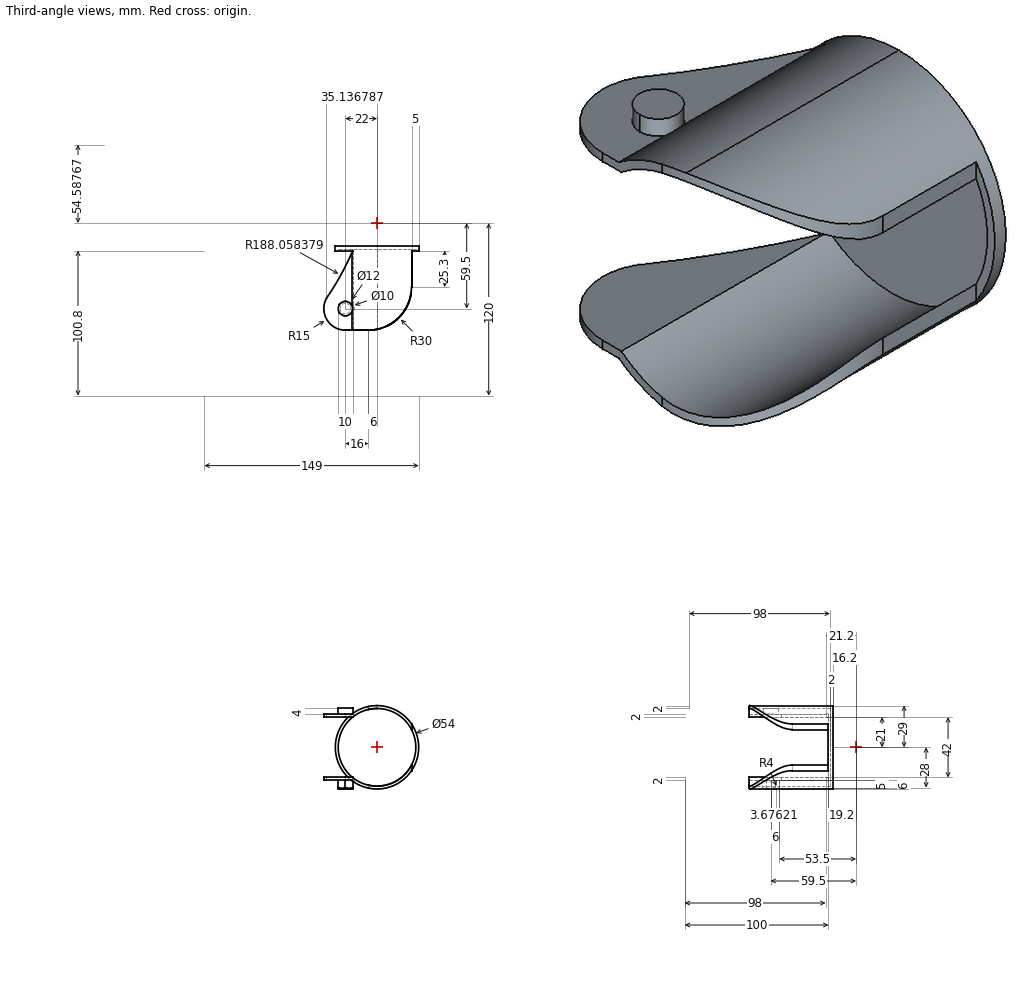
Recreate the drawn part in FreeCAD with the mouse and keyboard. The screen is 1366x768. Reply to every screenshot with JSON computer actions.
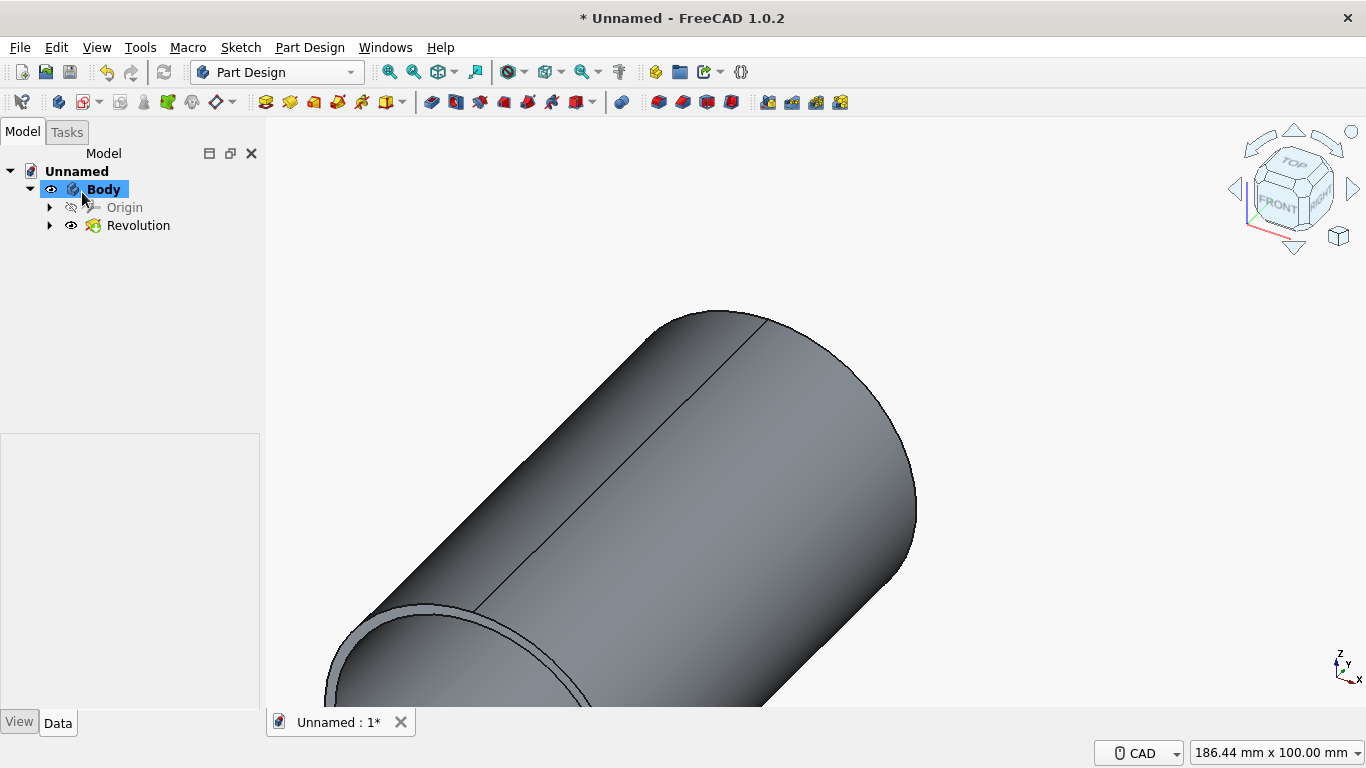
{"action": "key", "text": "v f"}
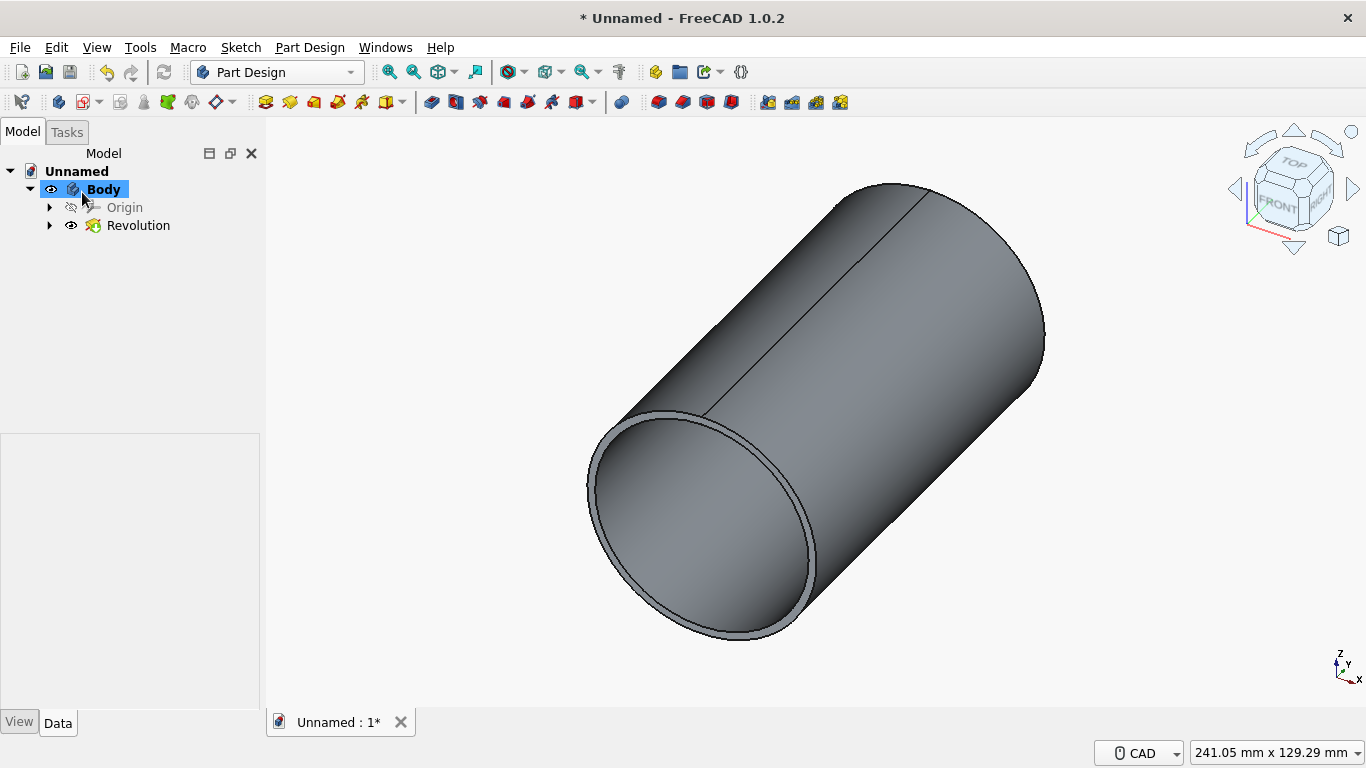
{"action": "left_click", "coordinate": [84, 102]}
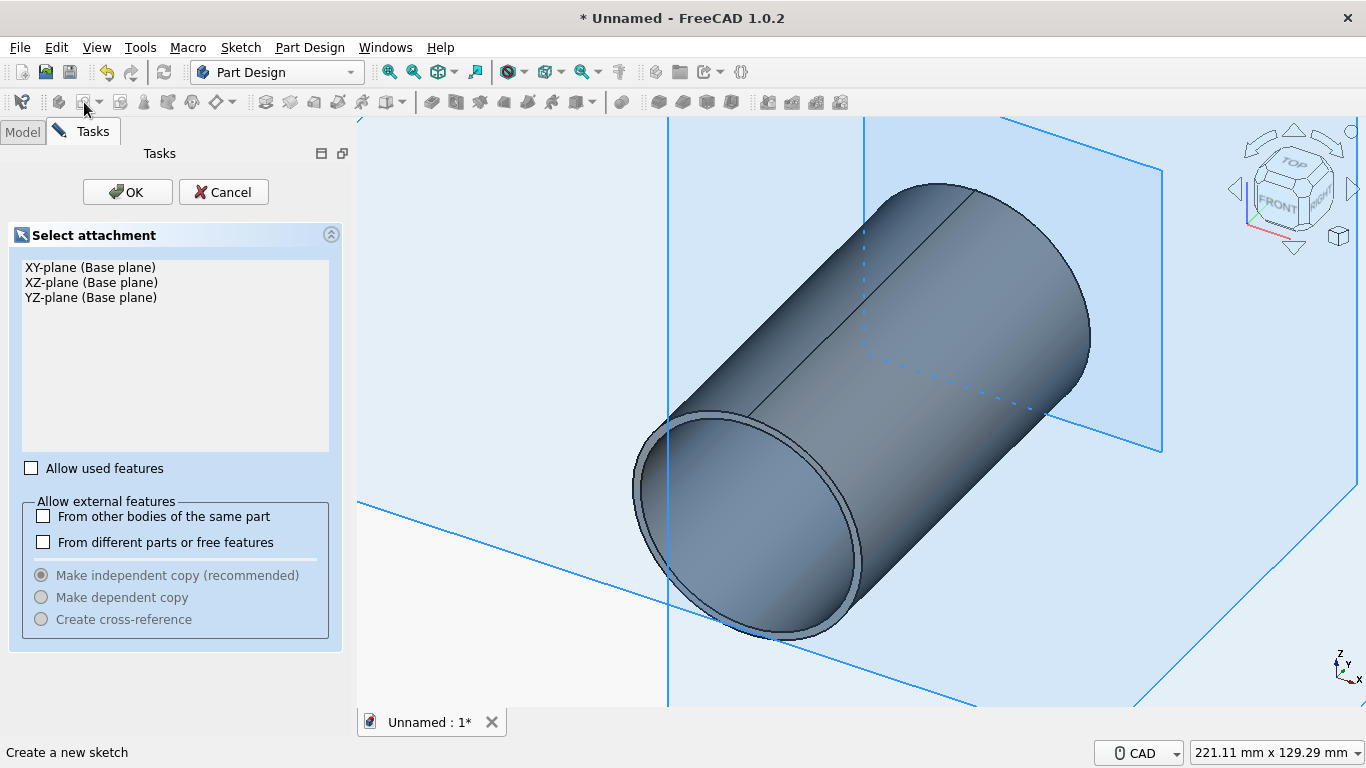
{"action": "left_click", "coordinate": [82, 298]}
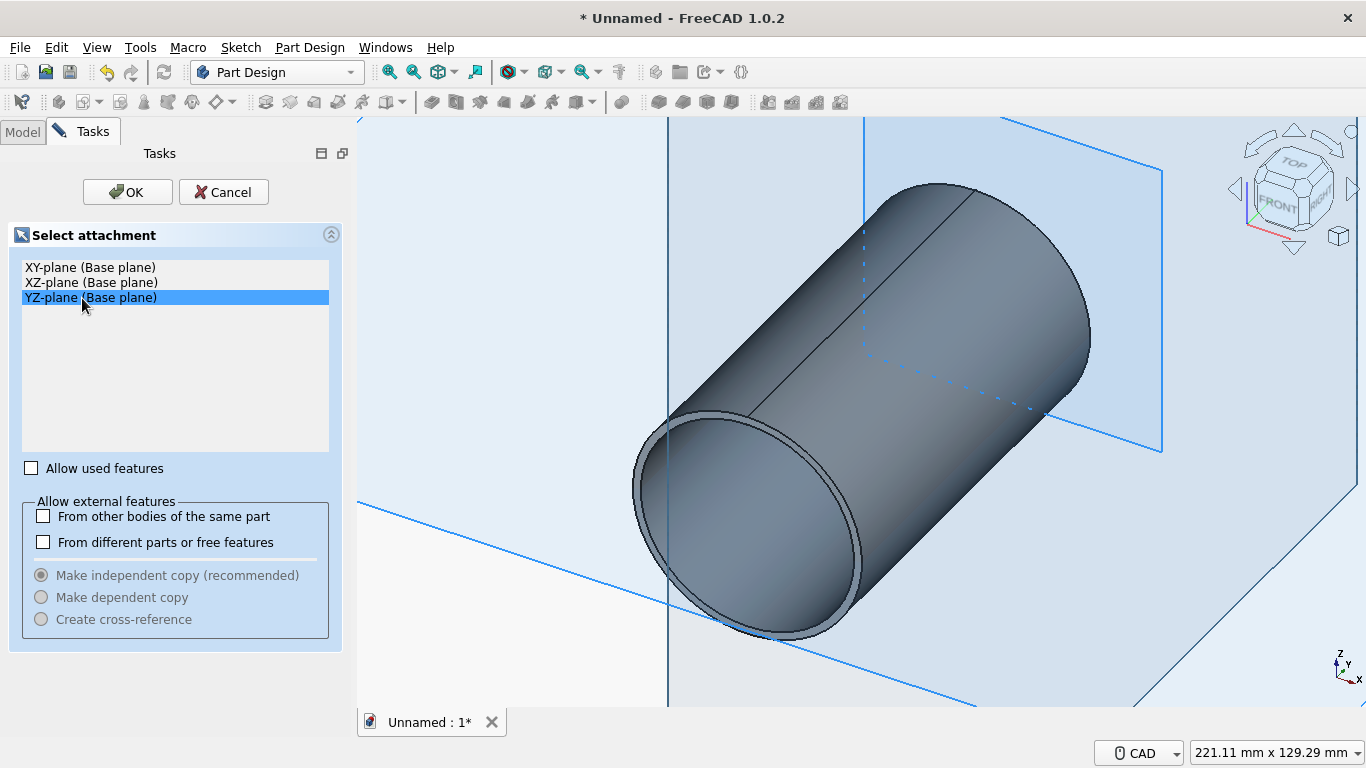
{"action": "left_click", "coordinate": [128, 192]}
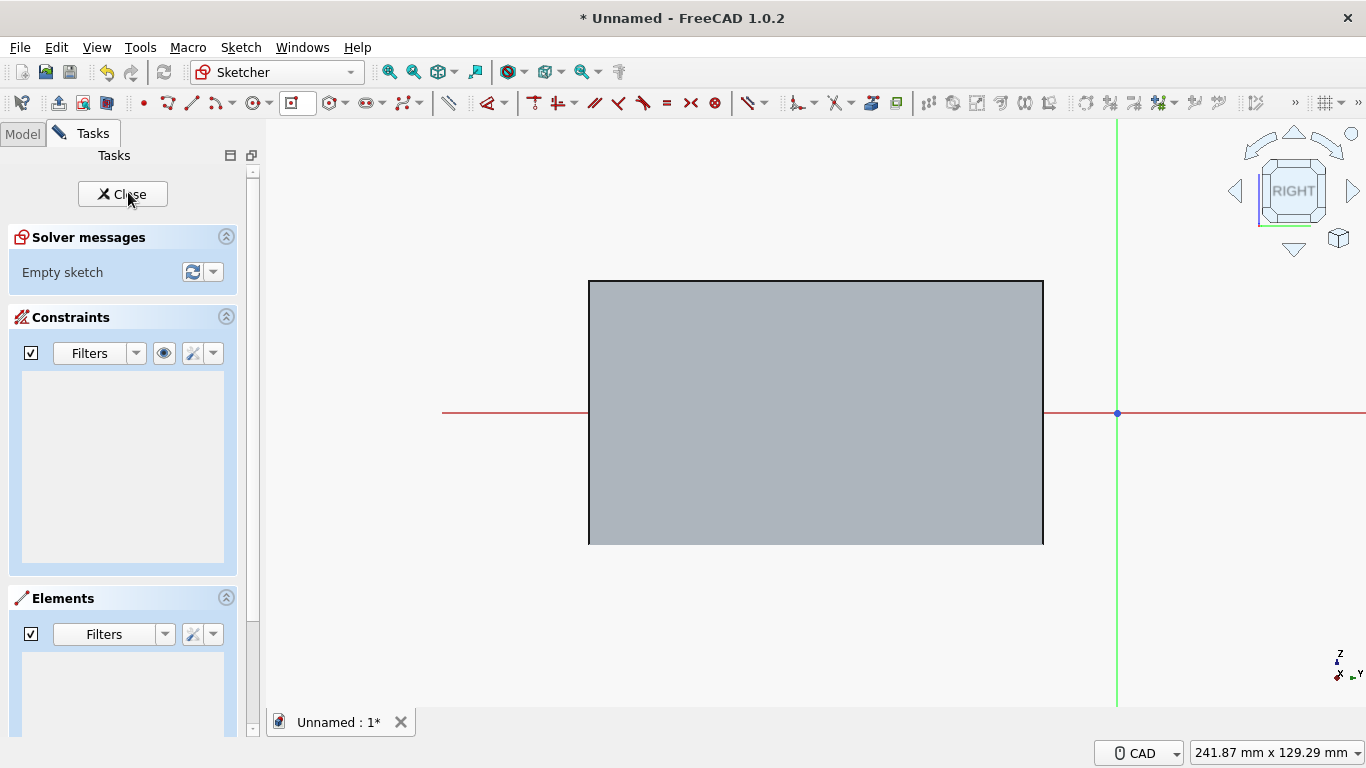
{"action": "key", "text": "q s"}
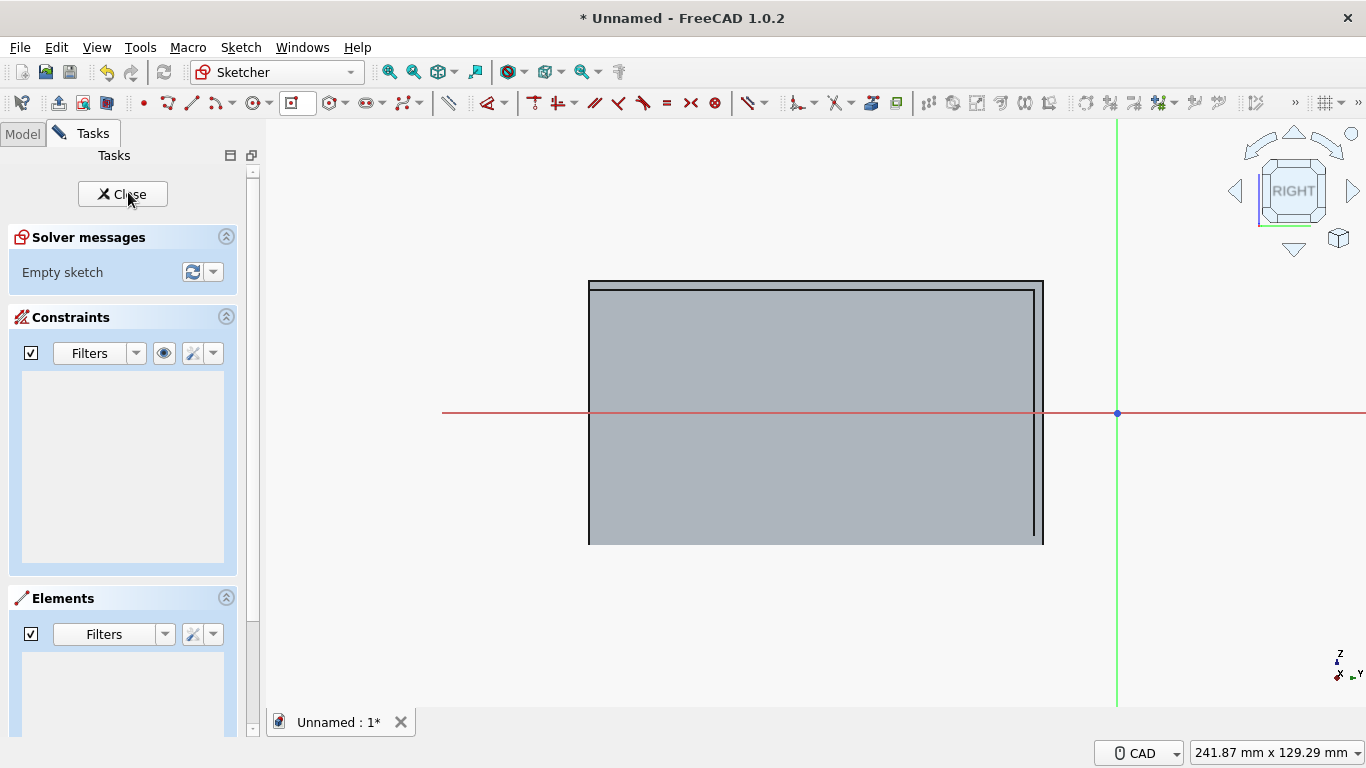
{"action": "key", "text": "g m"}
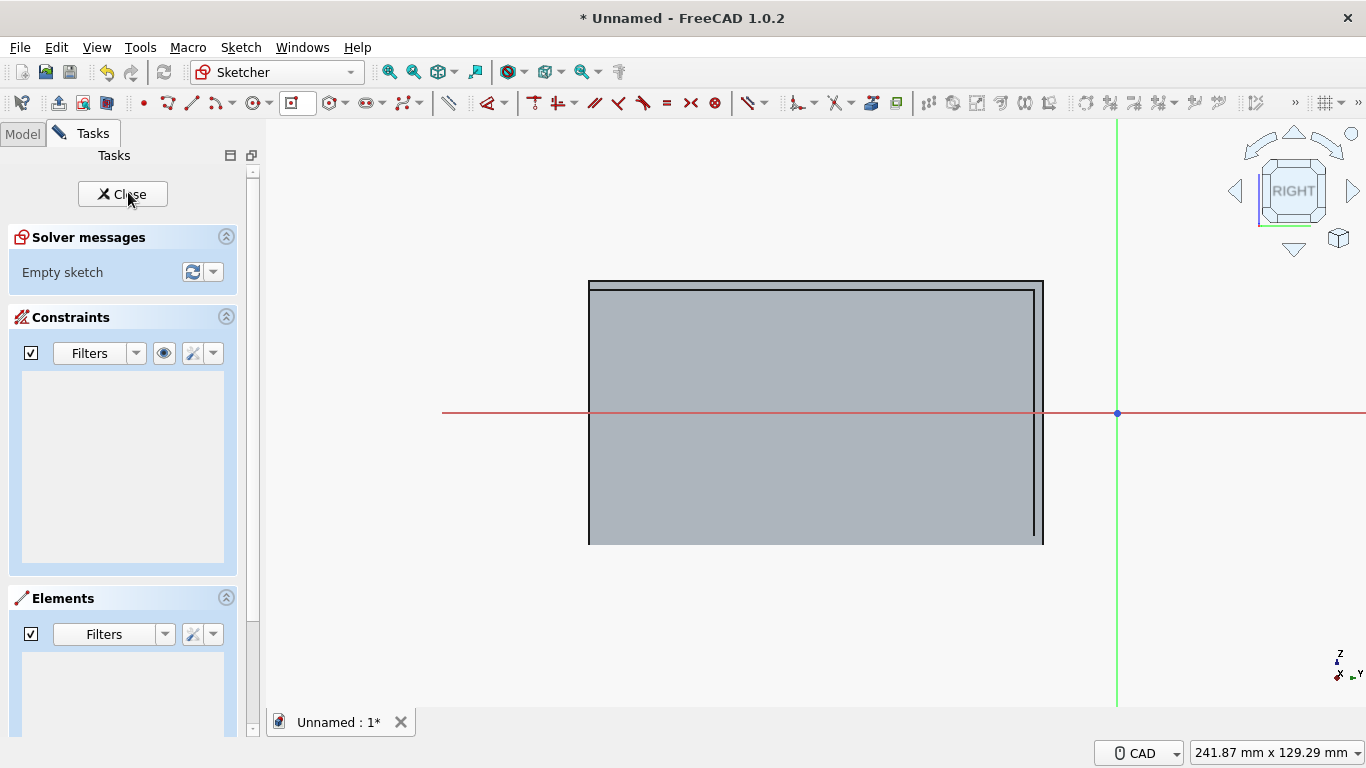
{"action": "left_click", "coordinate": [1021, 318]}
{"action": "left_click", "coordinate": [1021, 509]}
{"action": "left_click", "coordinate": [575, 509]}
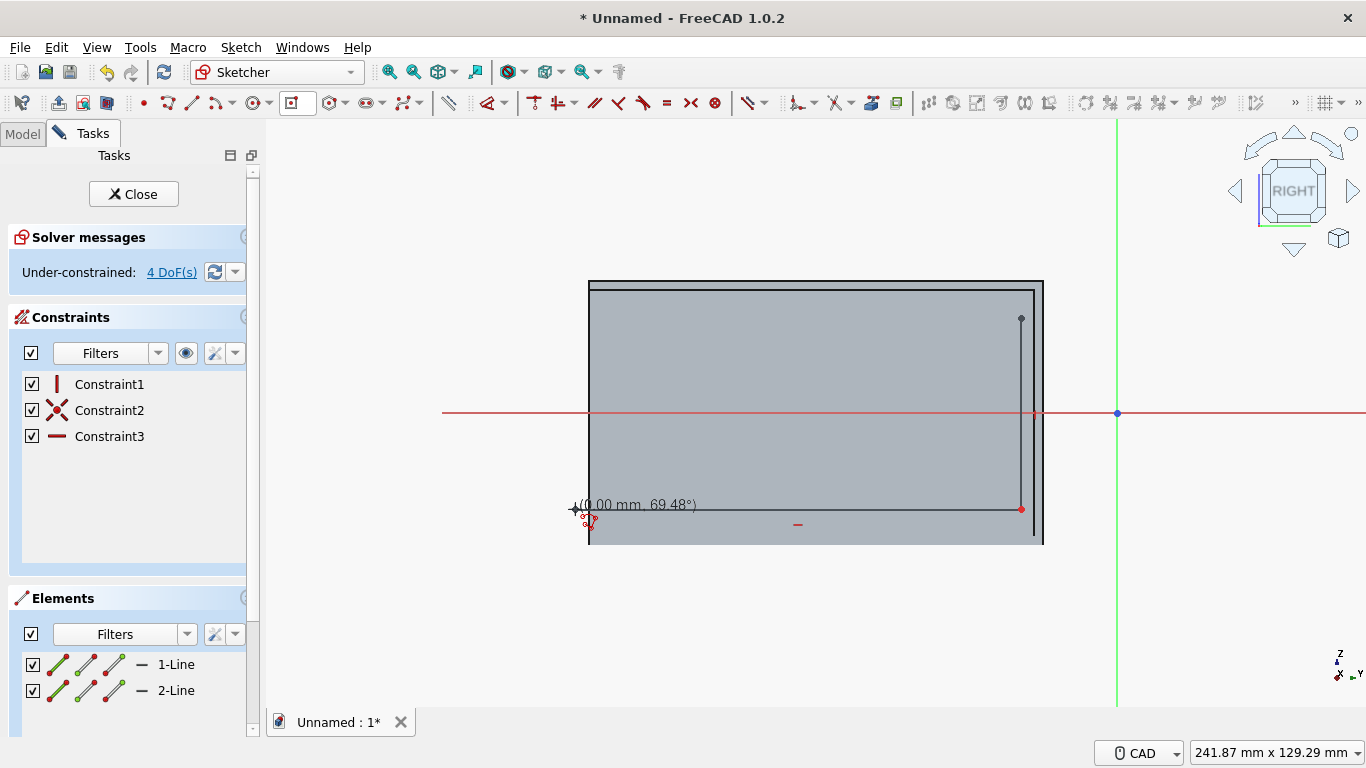
{"action": "scroll", "coordinate": [575, 518], "scroll_direction": "up", "scroll_amount": 3}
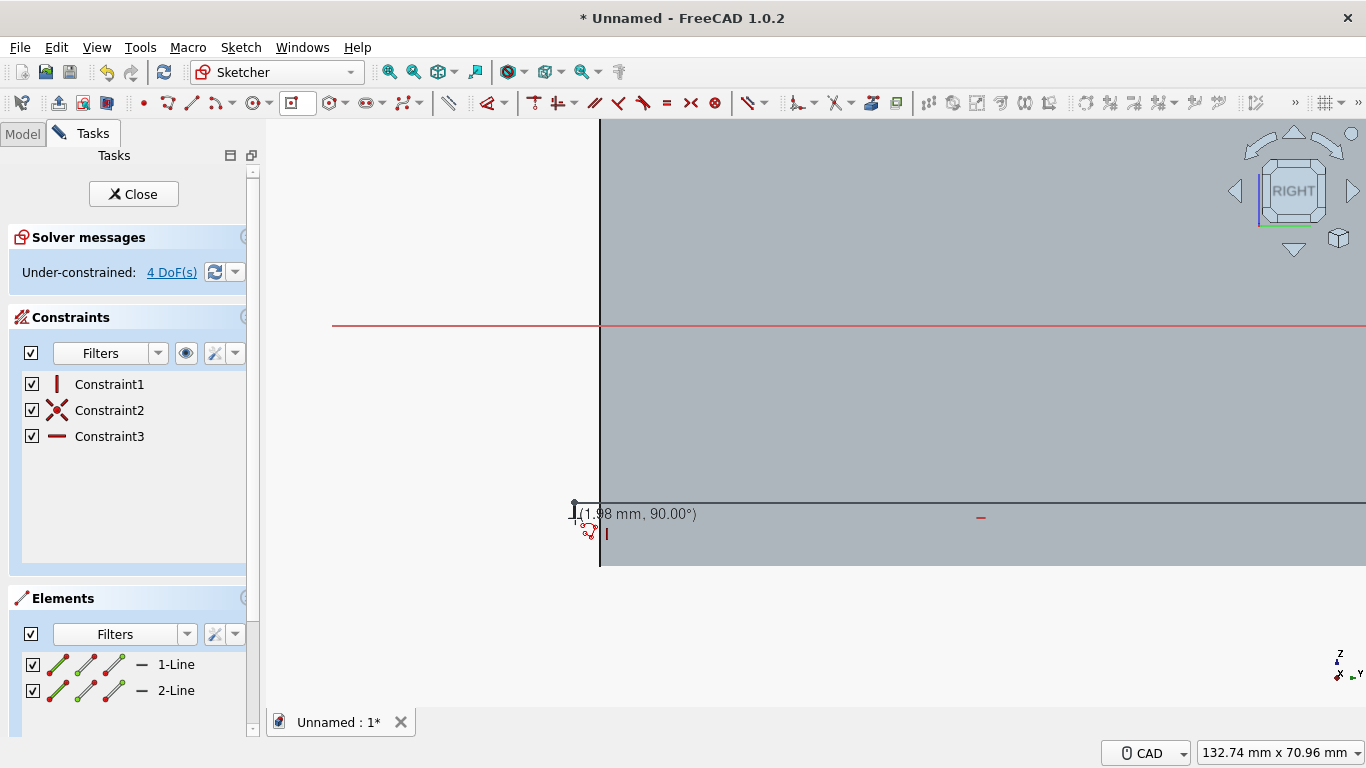
{"action": "left_click", "coordinate": [575, 517]}